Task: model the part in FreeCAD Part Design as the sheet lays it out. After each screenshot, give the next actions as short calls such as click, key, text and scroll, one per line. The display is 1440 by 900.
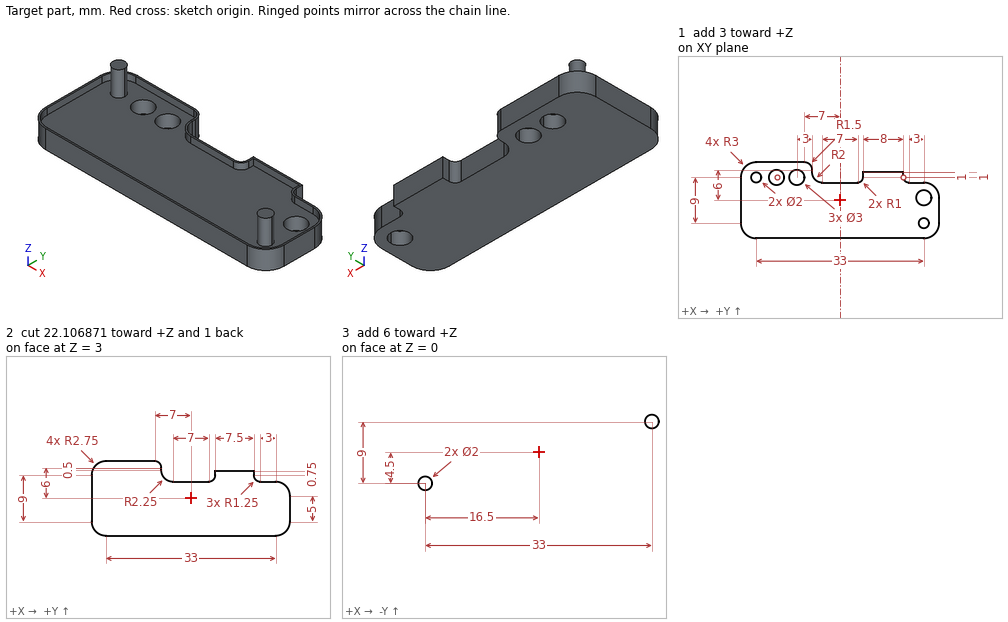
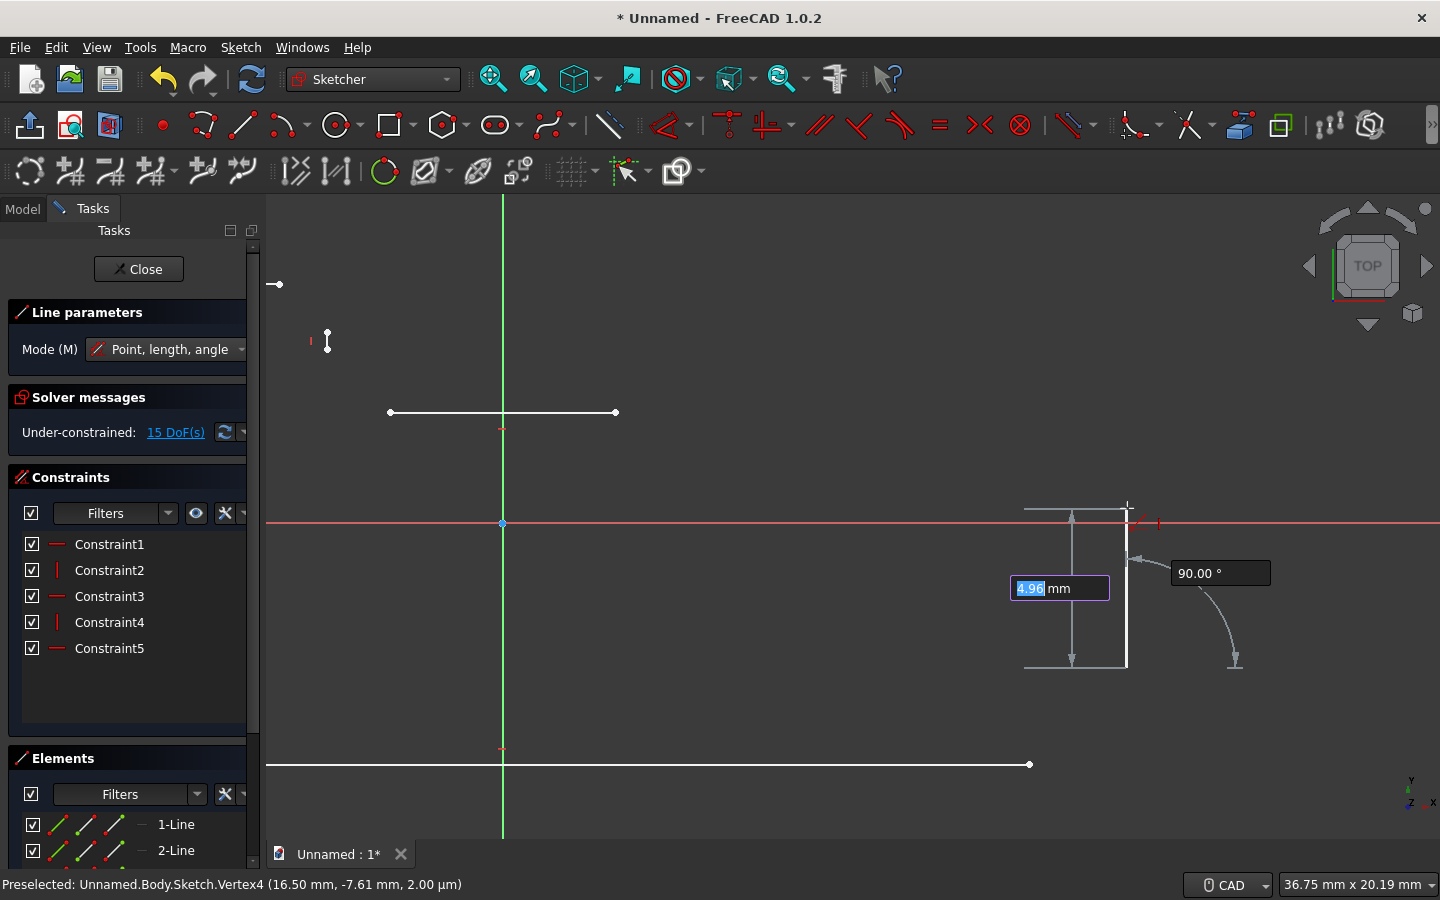
click(1126, 507)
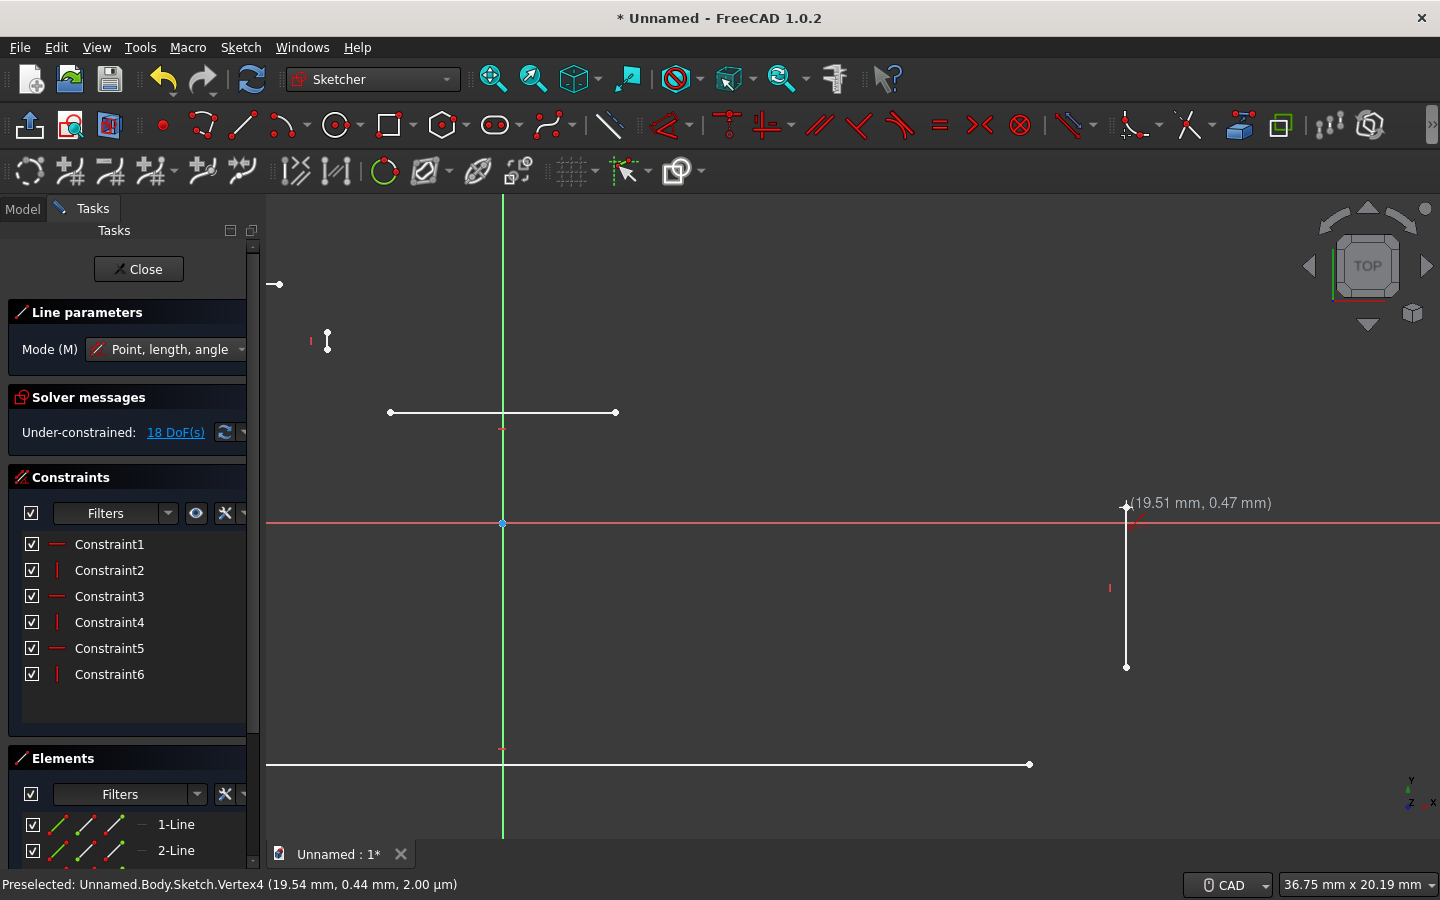
click(1030, 411)
click(934, 411)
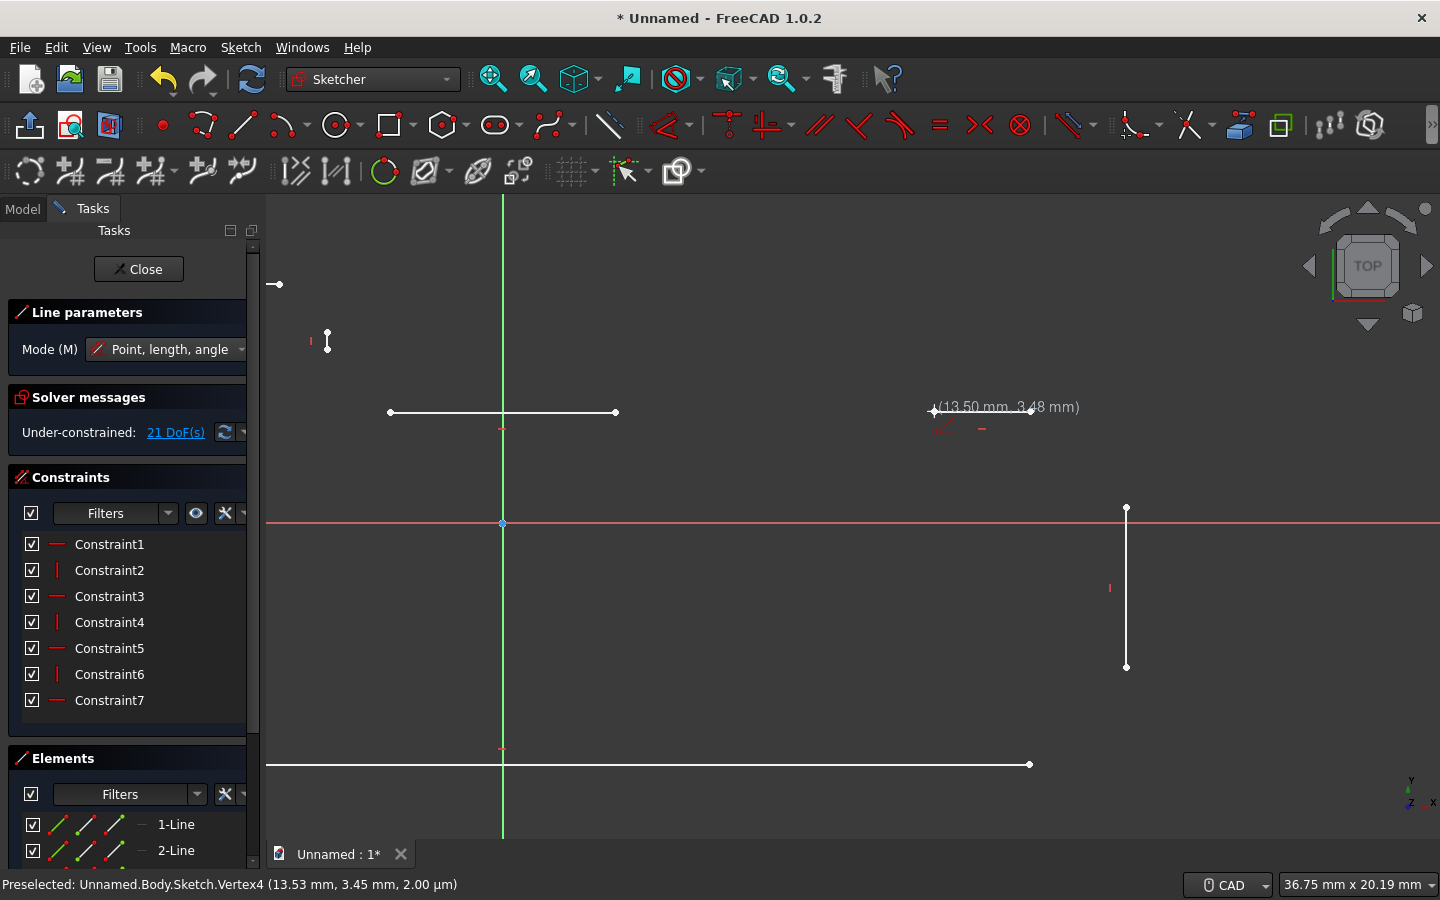
key(g)
key(m)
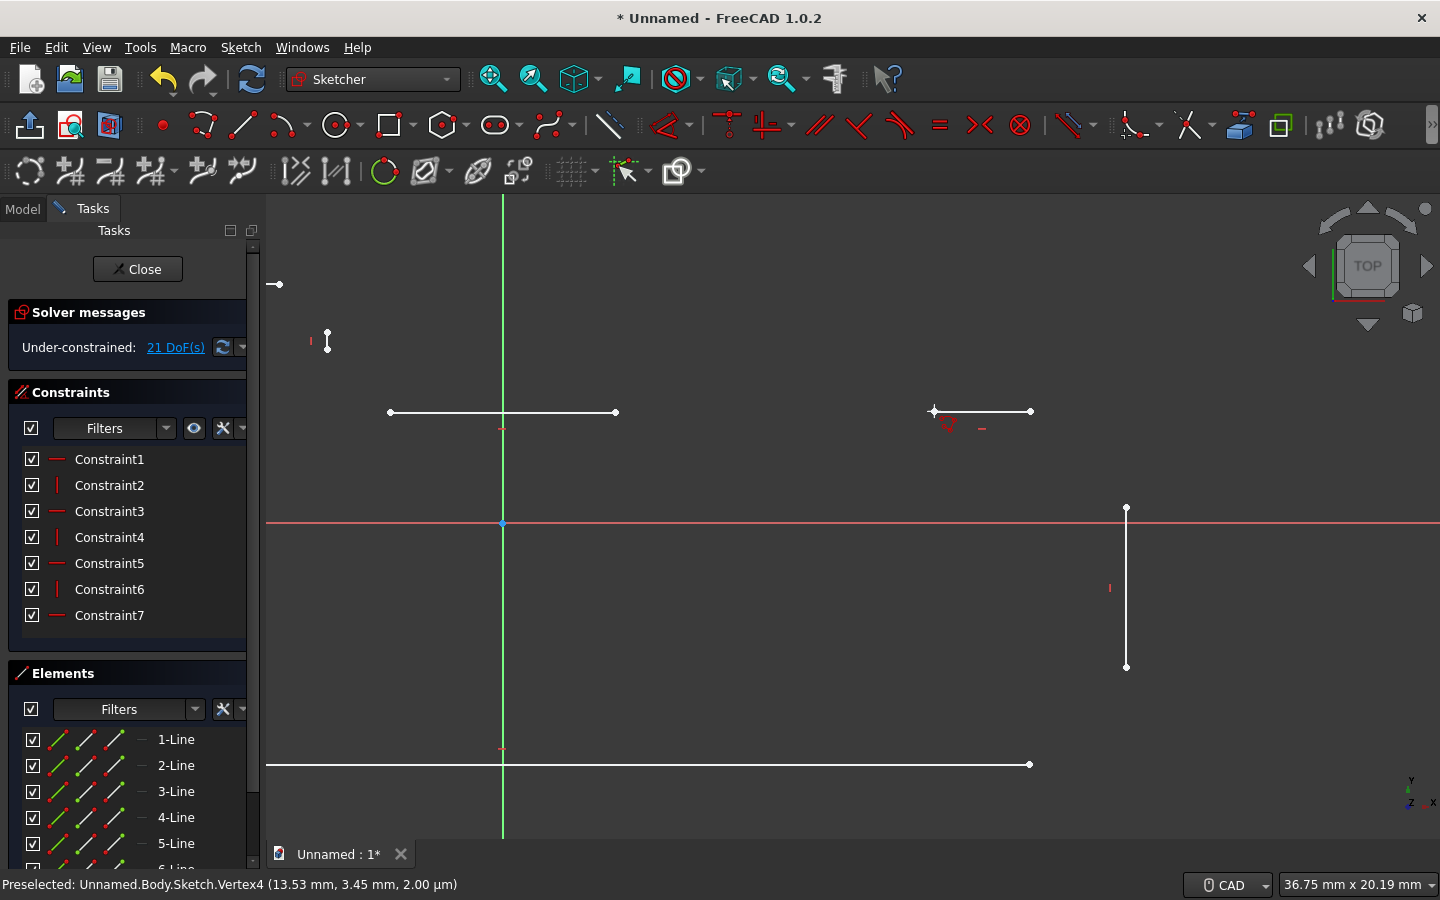
click(902, 379)
click(902, 347)
click(646, 347)
click(646, 379)
right_click(646, 379)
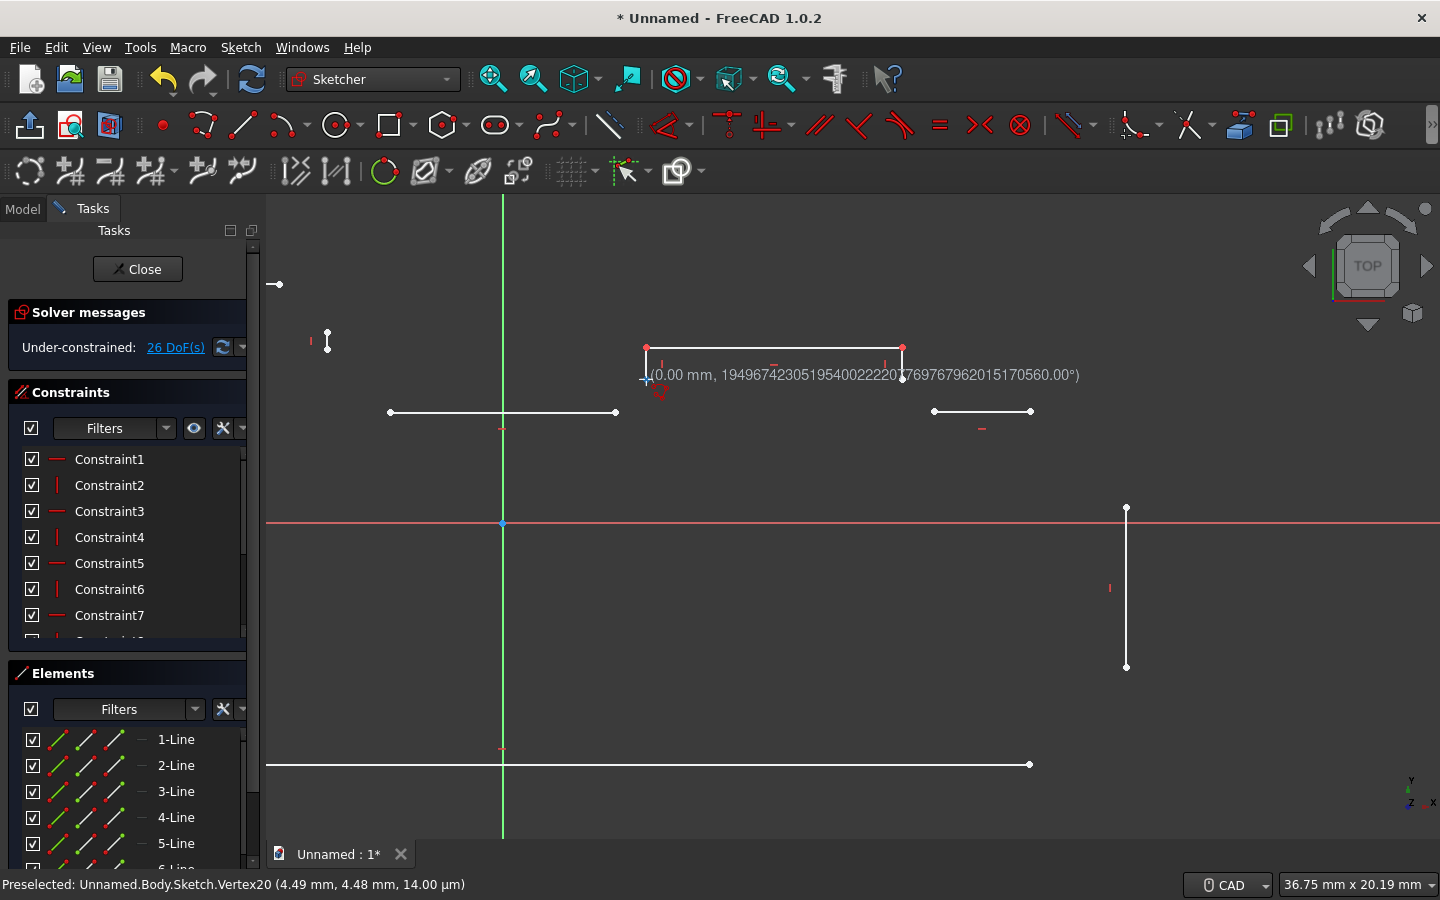
key(g)
key(3)
key(a)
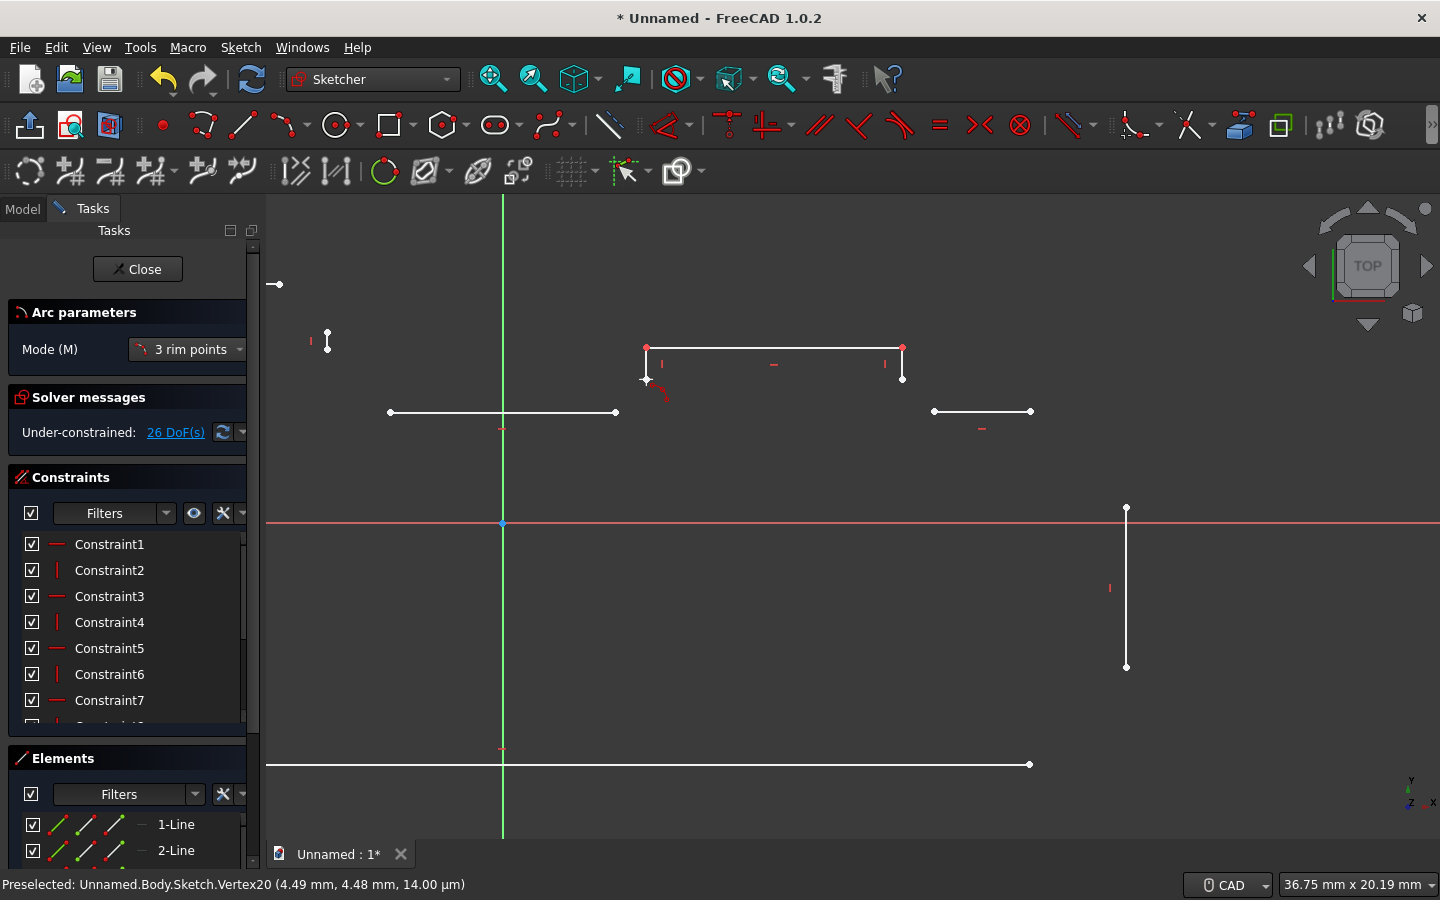
click(391, 413)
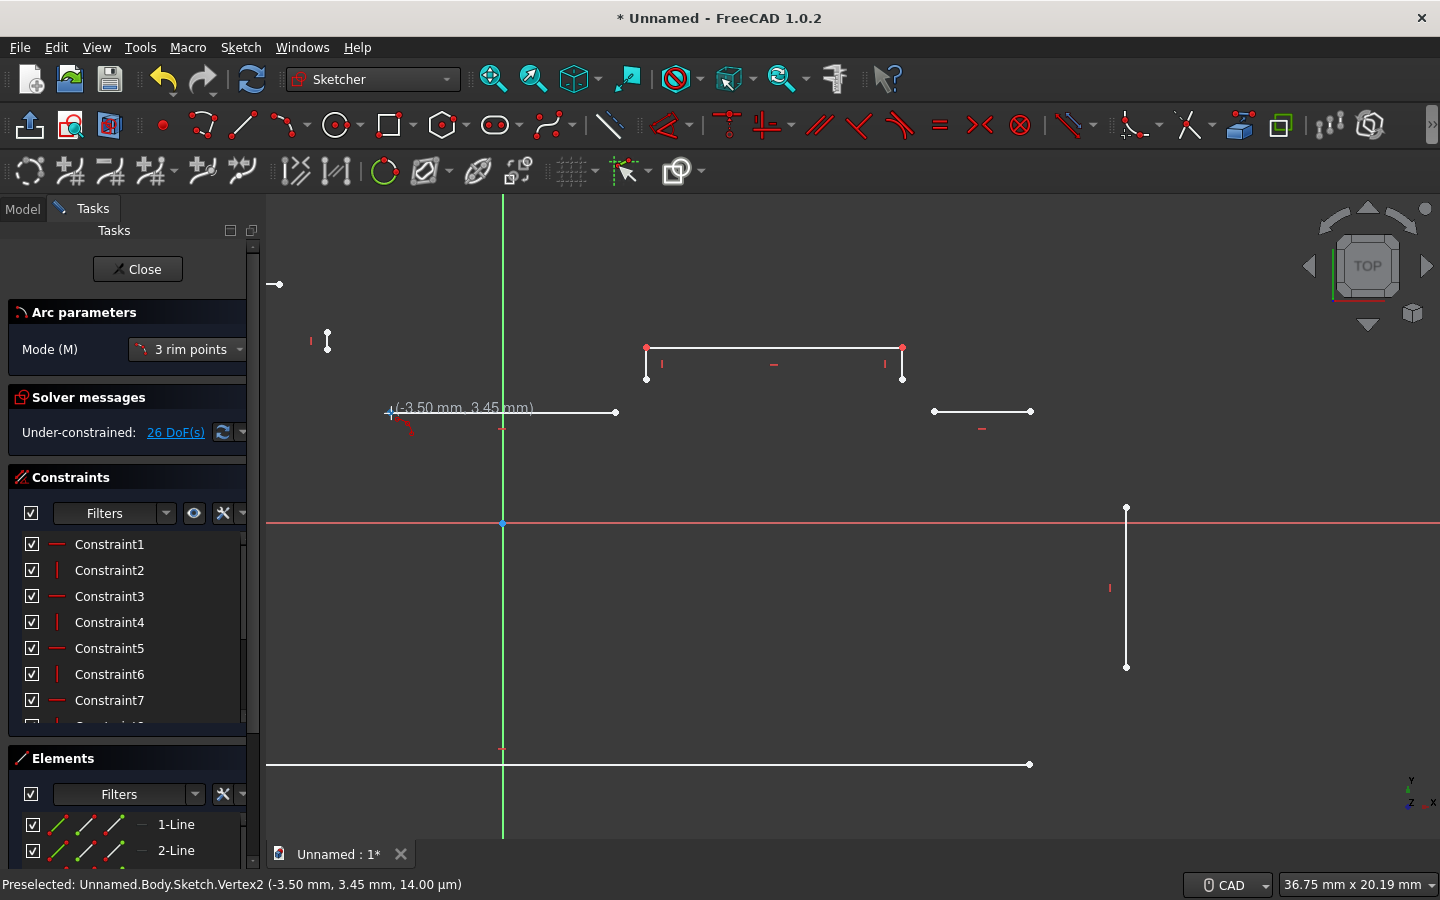
scroll(327, 347, up, 4)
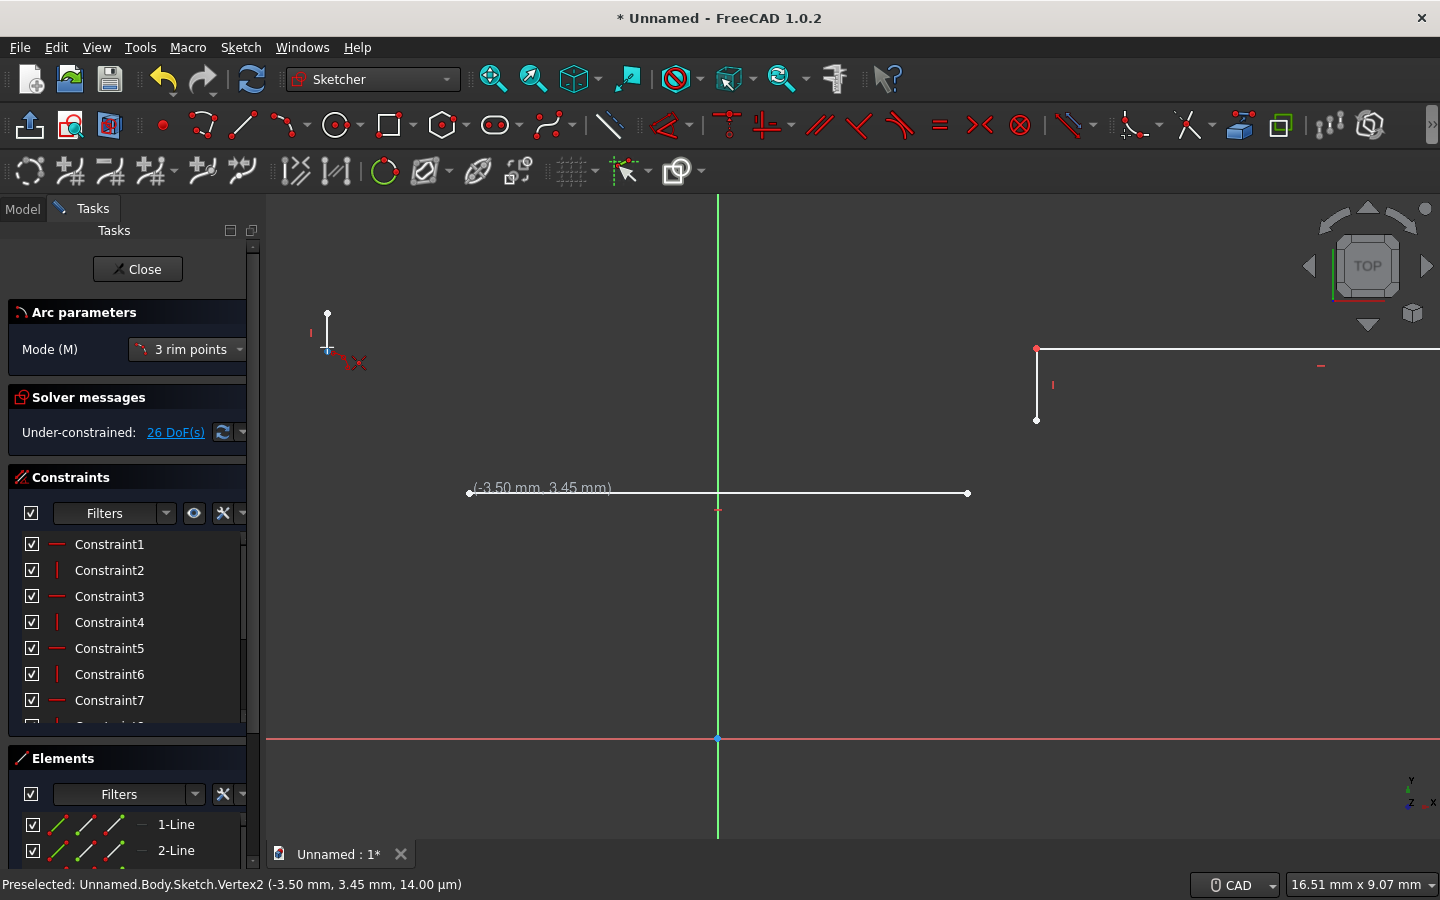
click(327, 351)
click(369, 448)